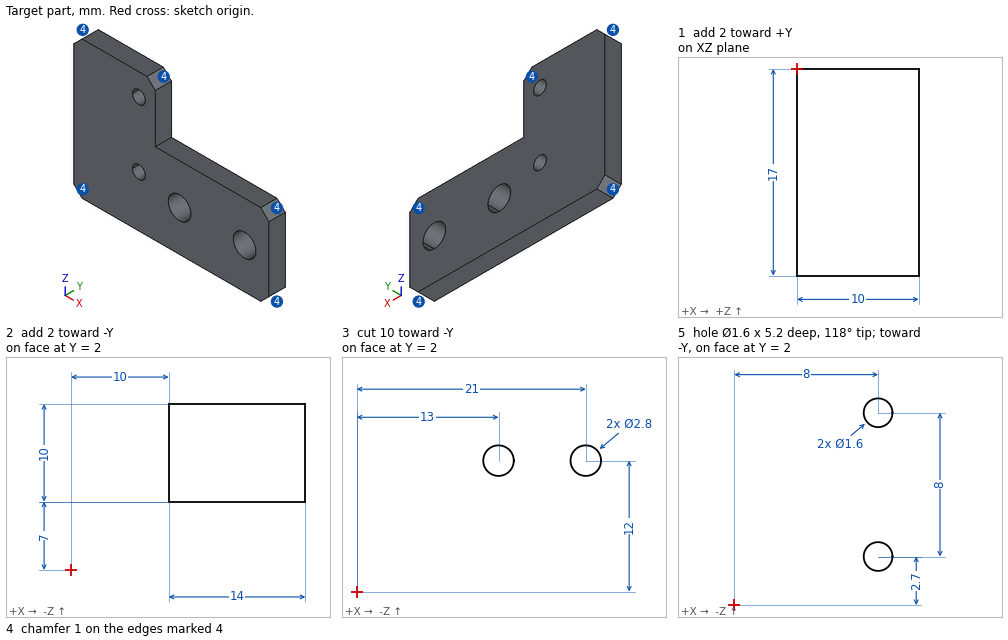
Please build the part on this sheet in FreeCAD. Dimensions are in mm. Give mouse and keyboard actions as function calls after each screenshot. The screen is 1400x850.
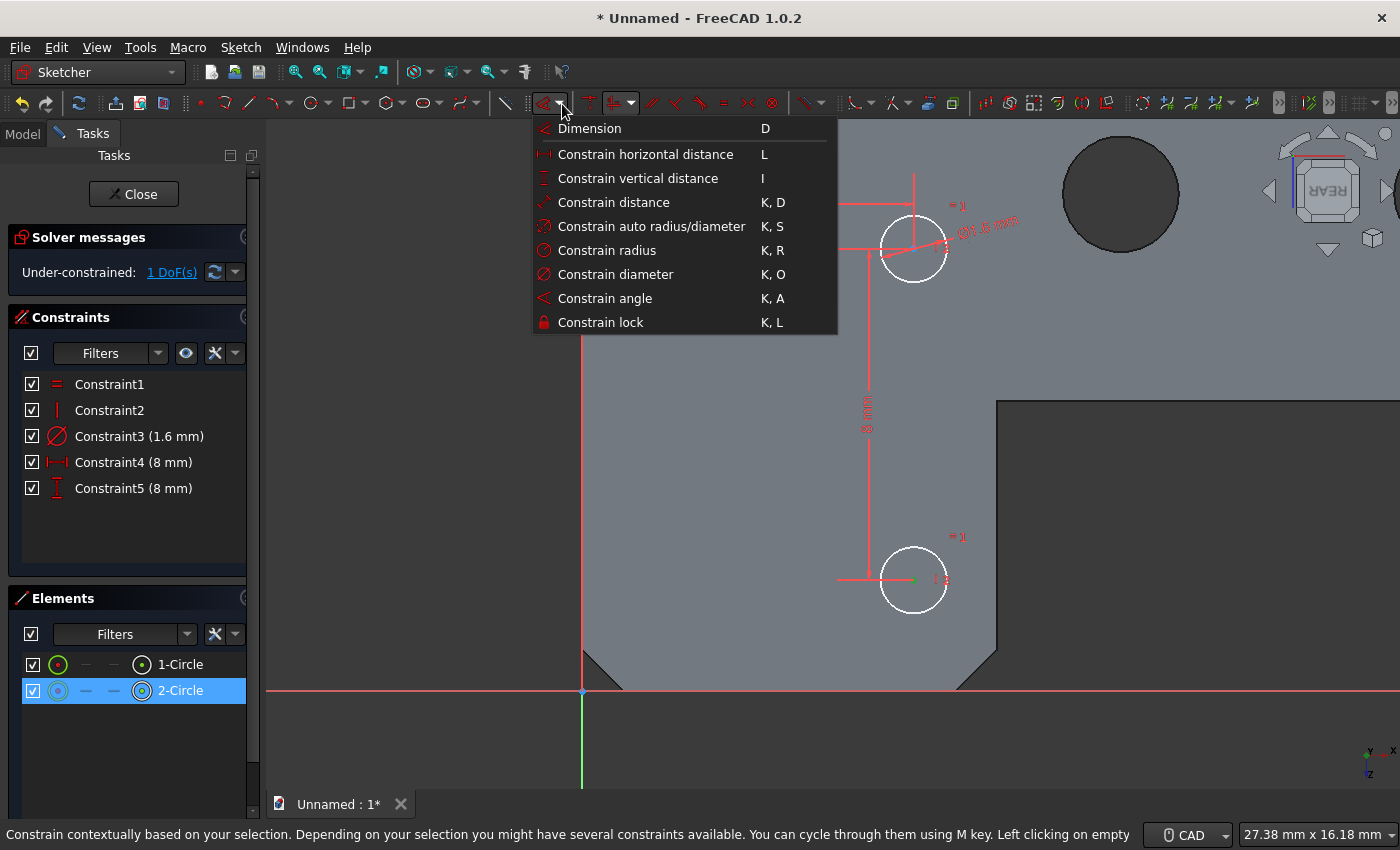
click(685, 178)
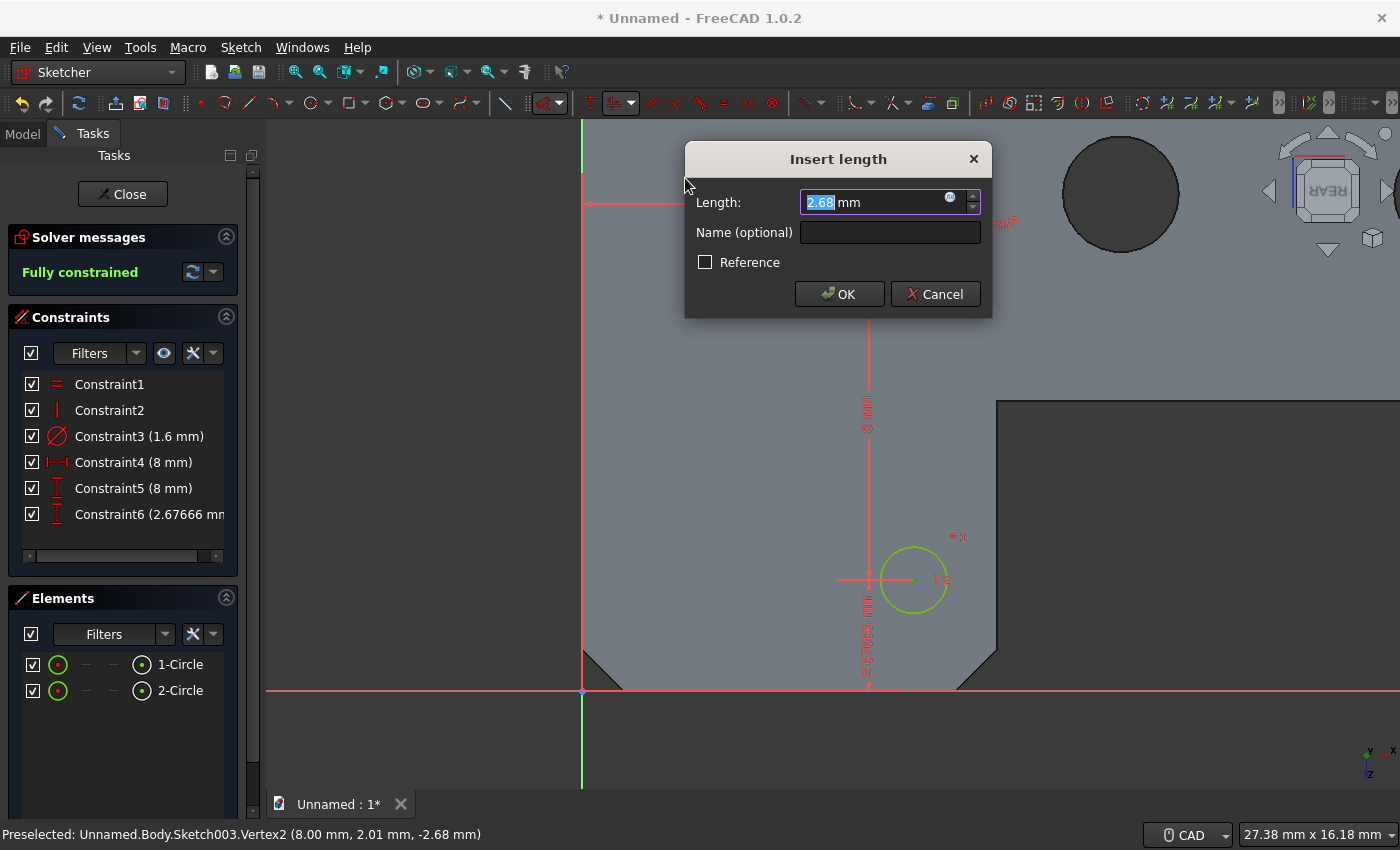
text(2.7)
key(Return)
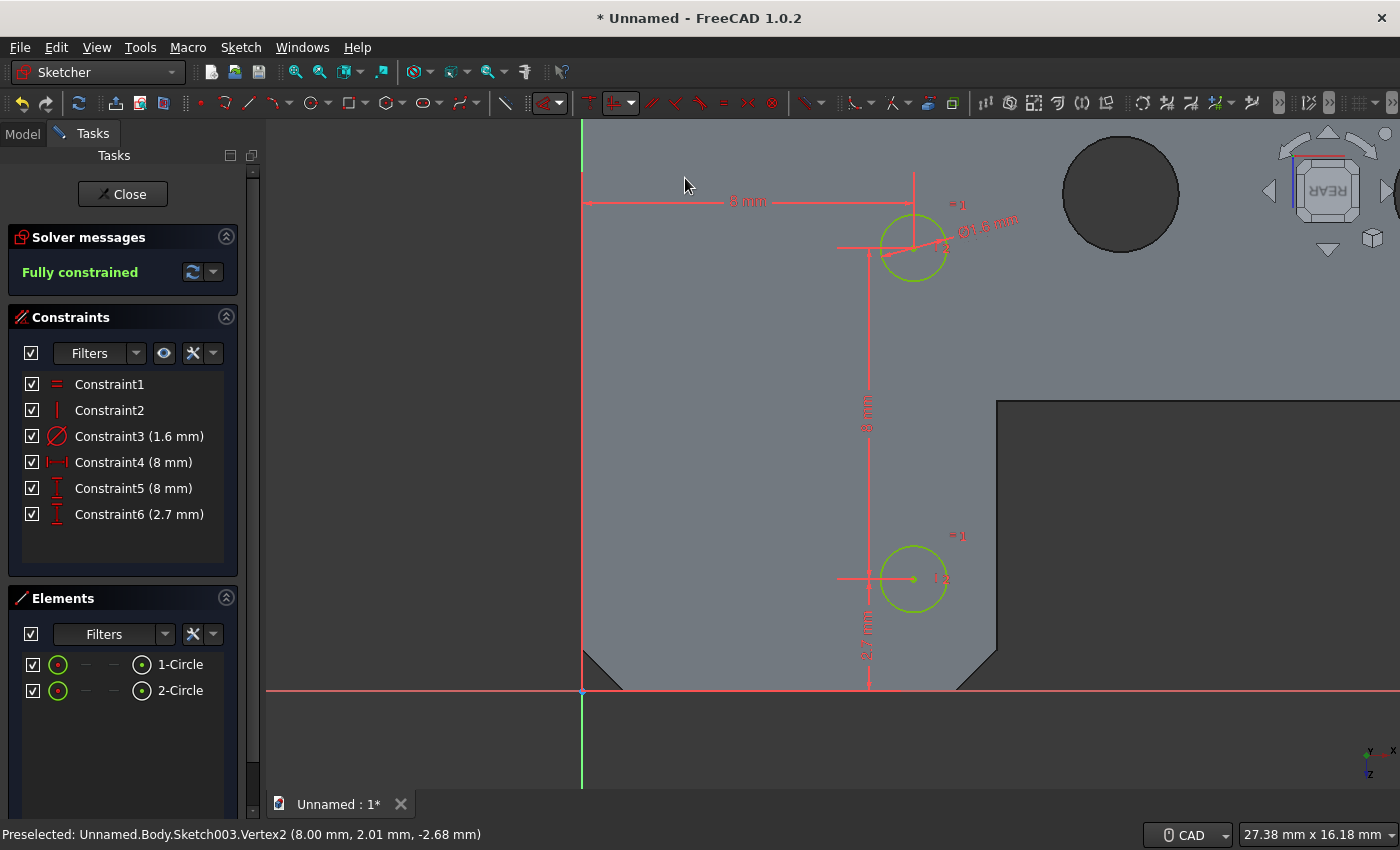
click(123, 194)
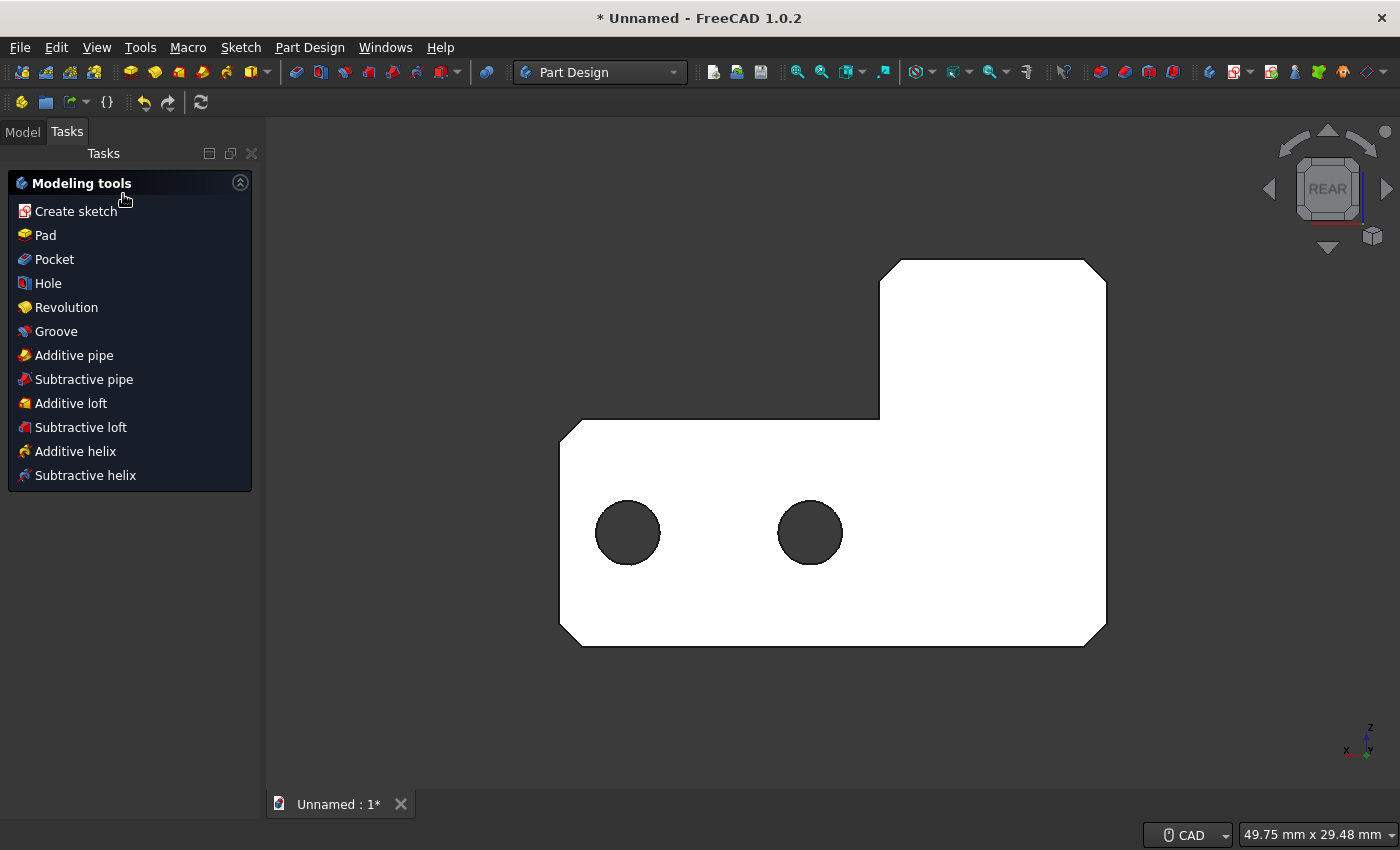
click(322, 72)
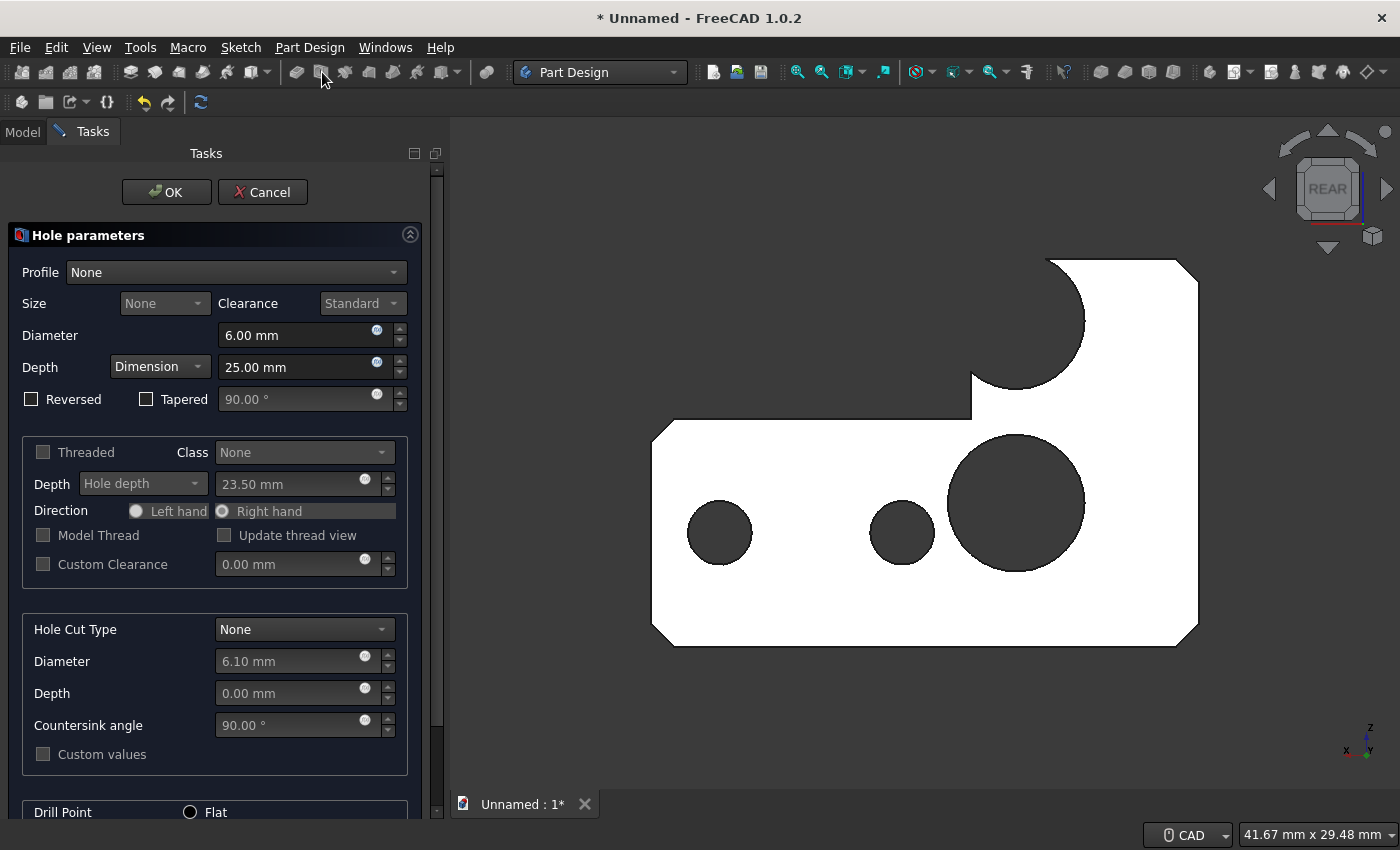
triple_click(305, 335)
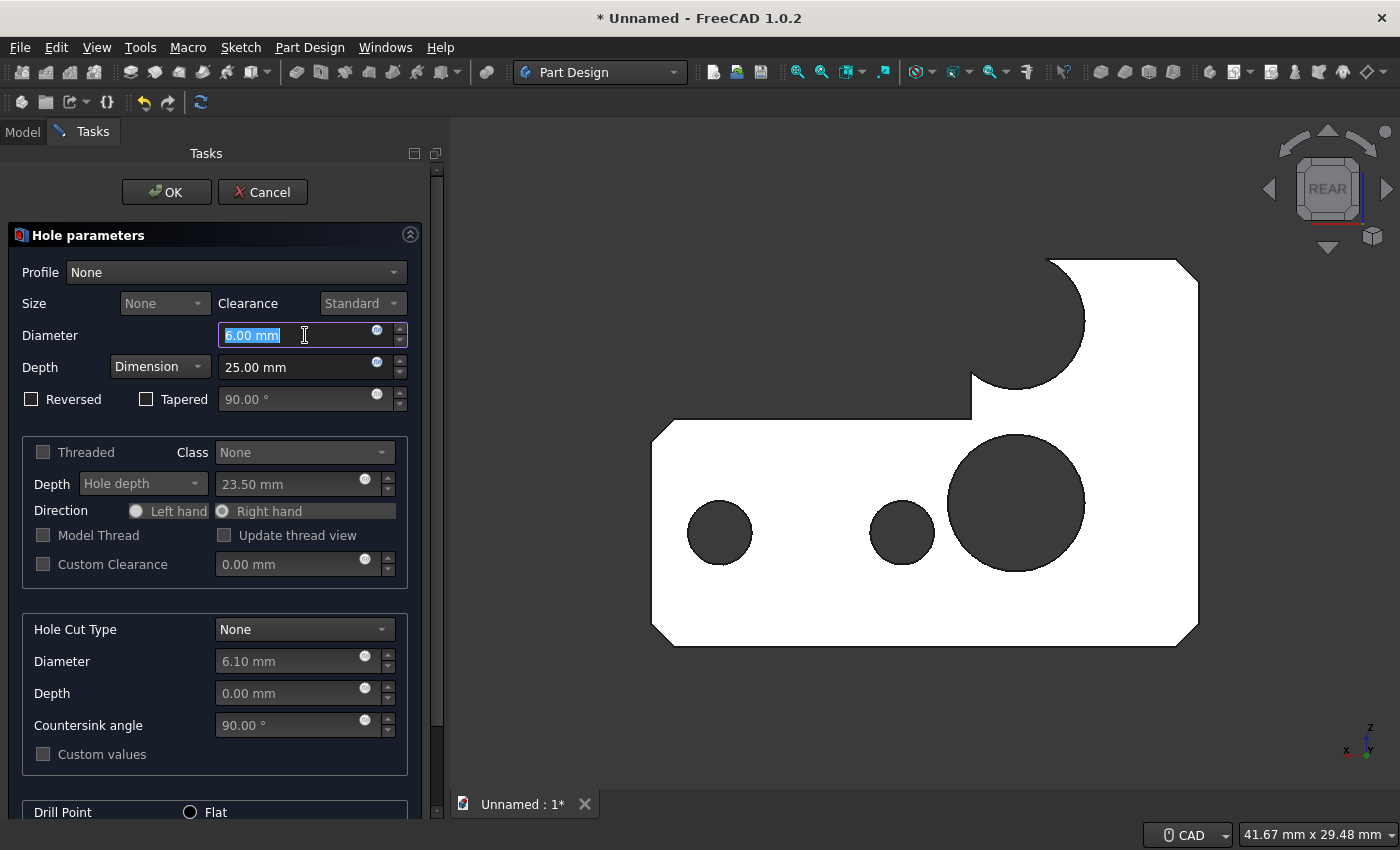
text(1.6)
key(Tab)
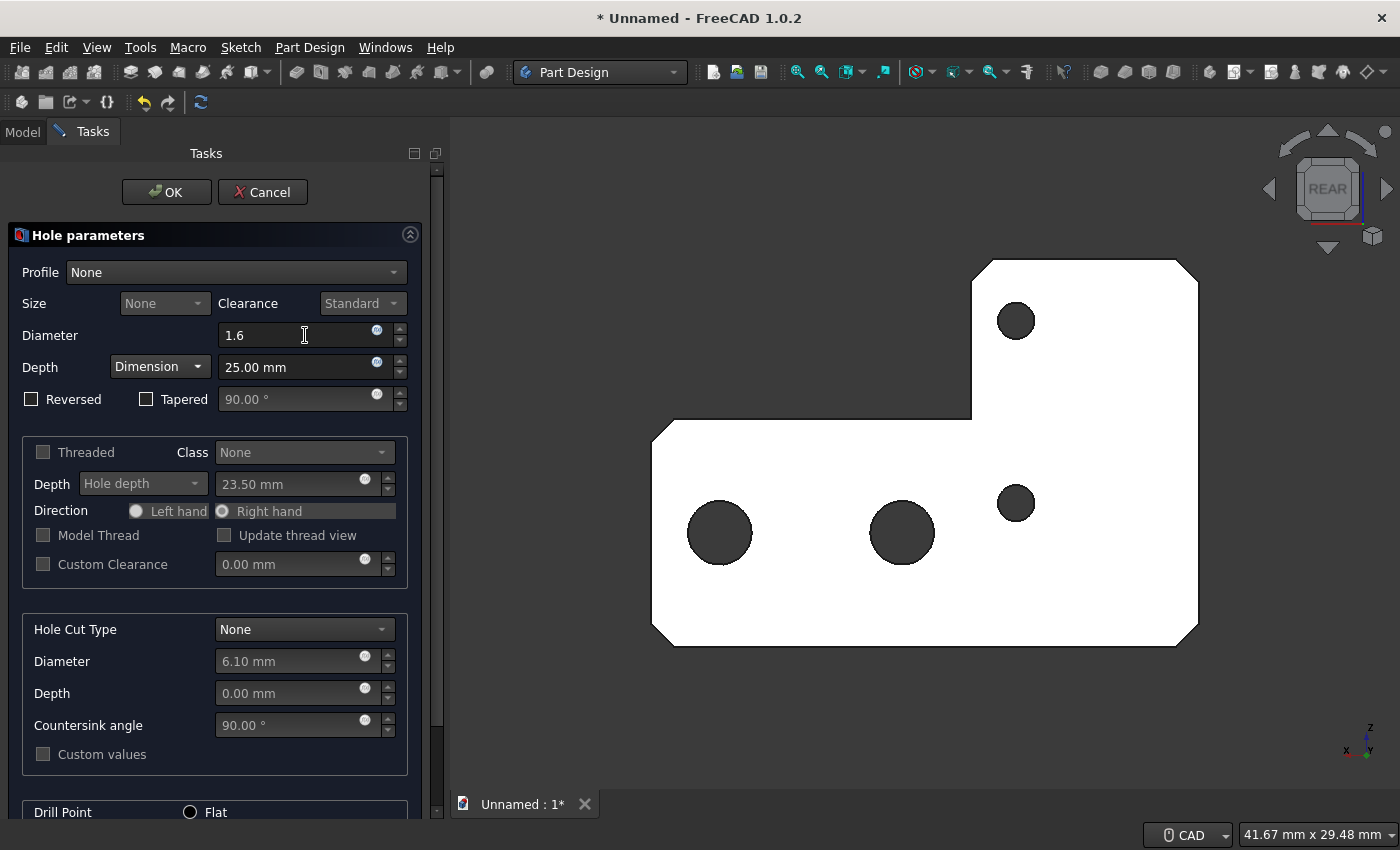
triple_click(305, 367)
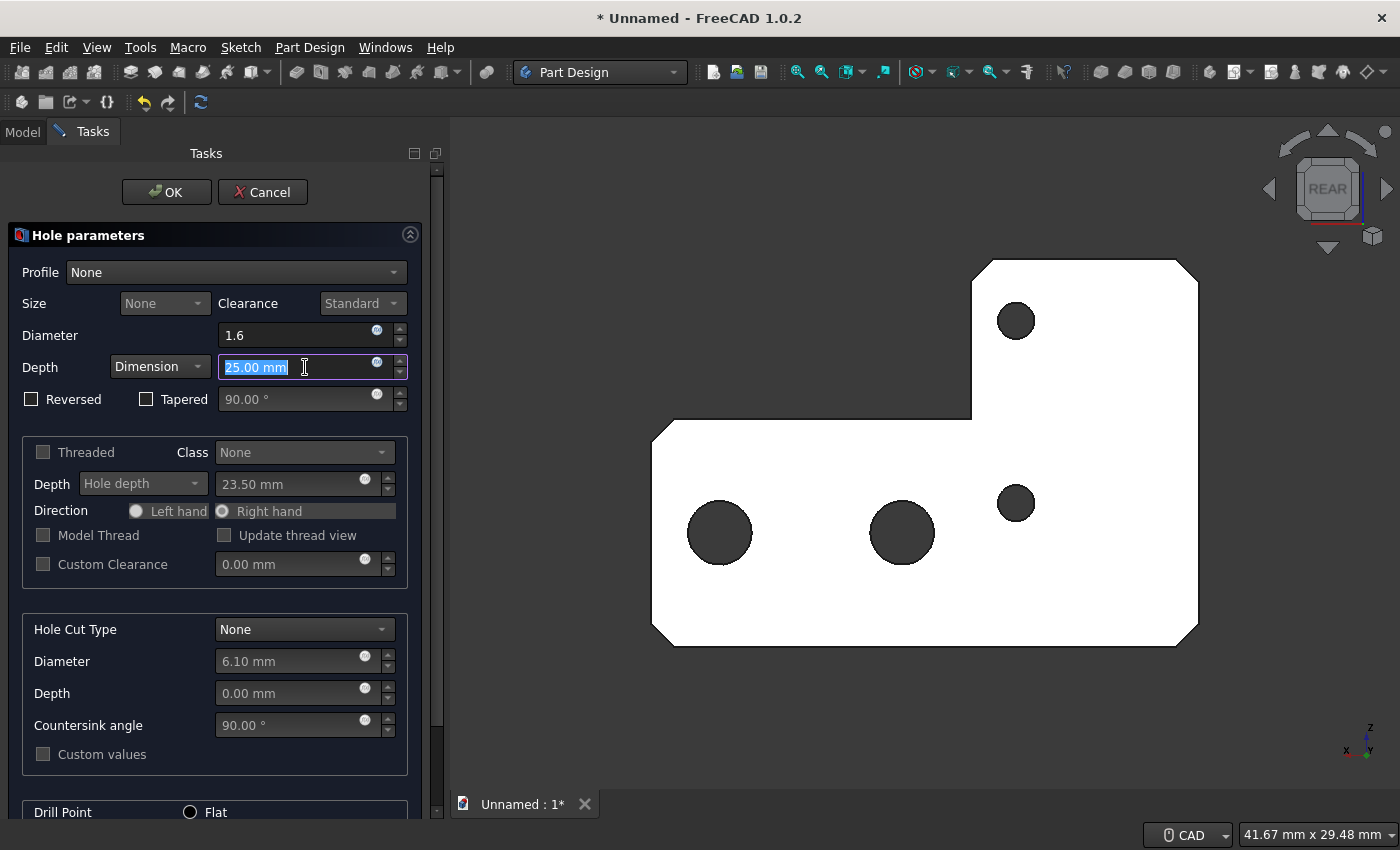
text(5.2)
key(Tab)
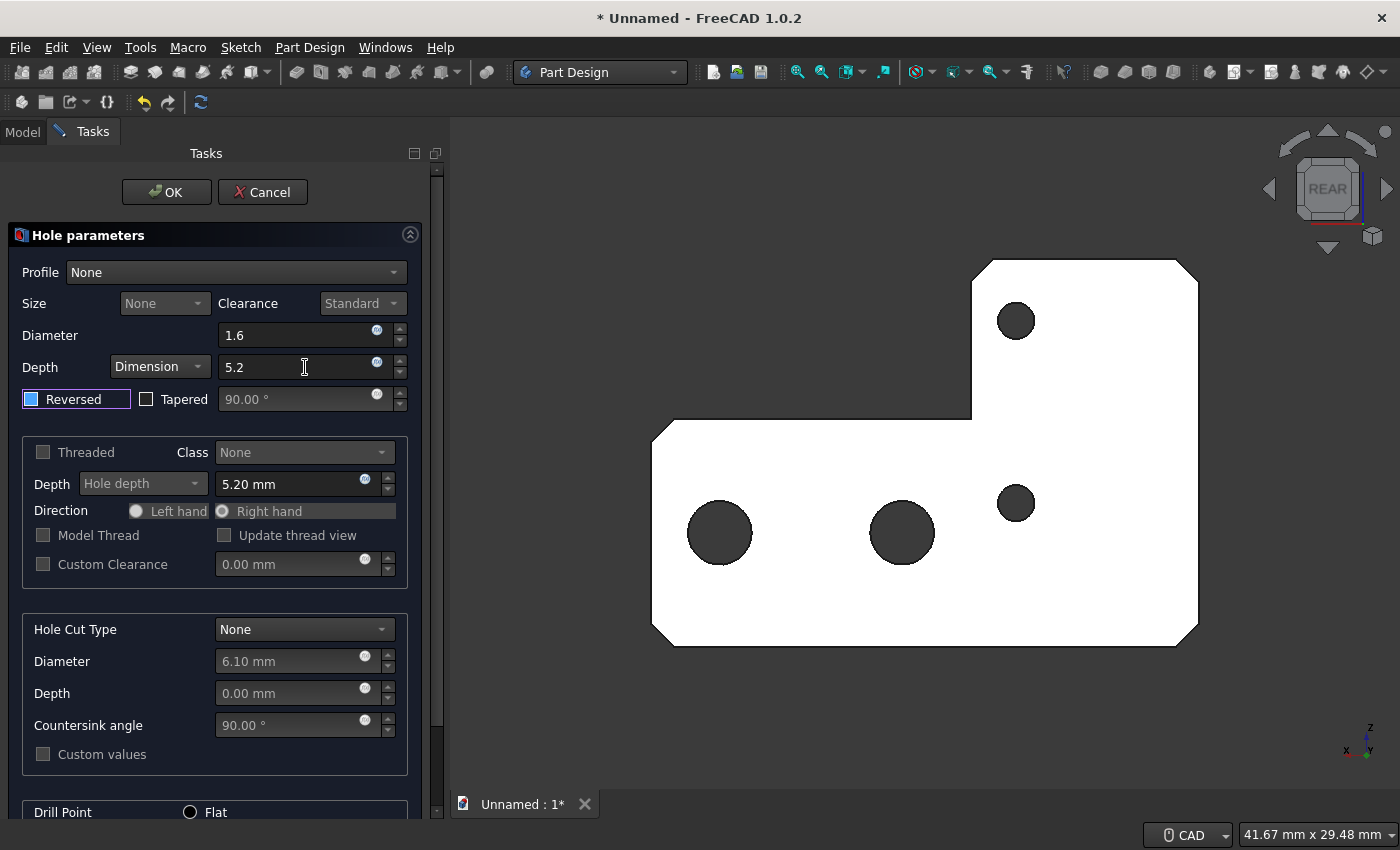
click(167, 192)